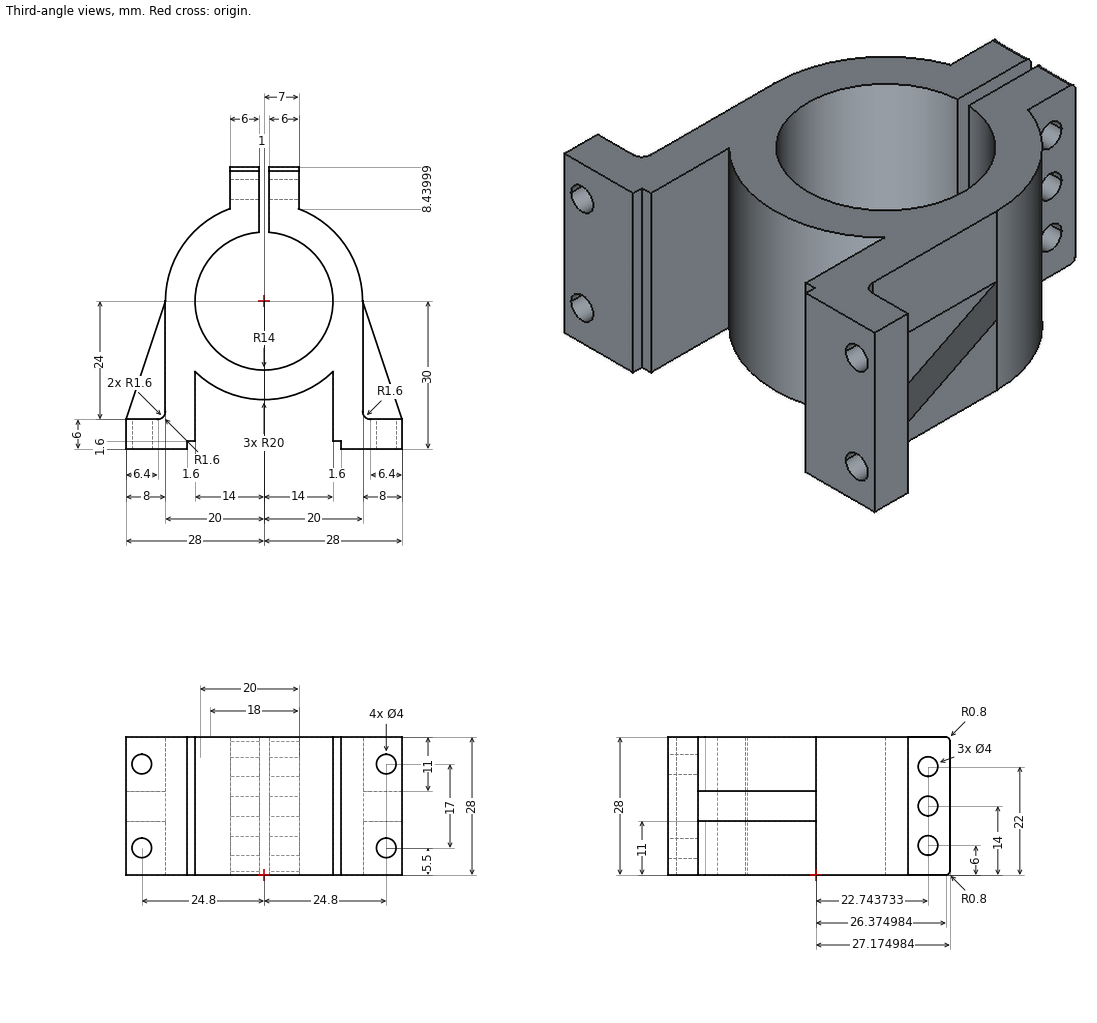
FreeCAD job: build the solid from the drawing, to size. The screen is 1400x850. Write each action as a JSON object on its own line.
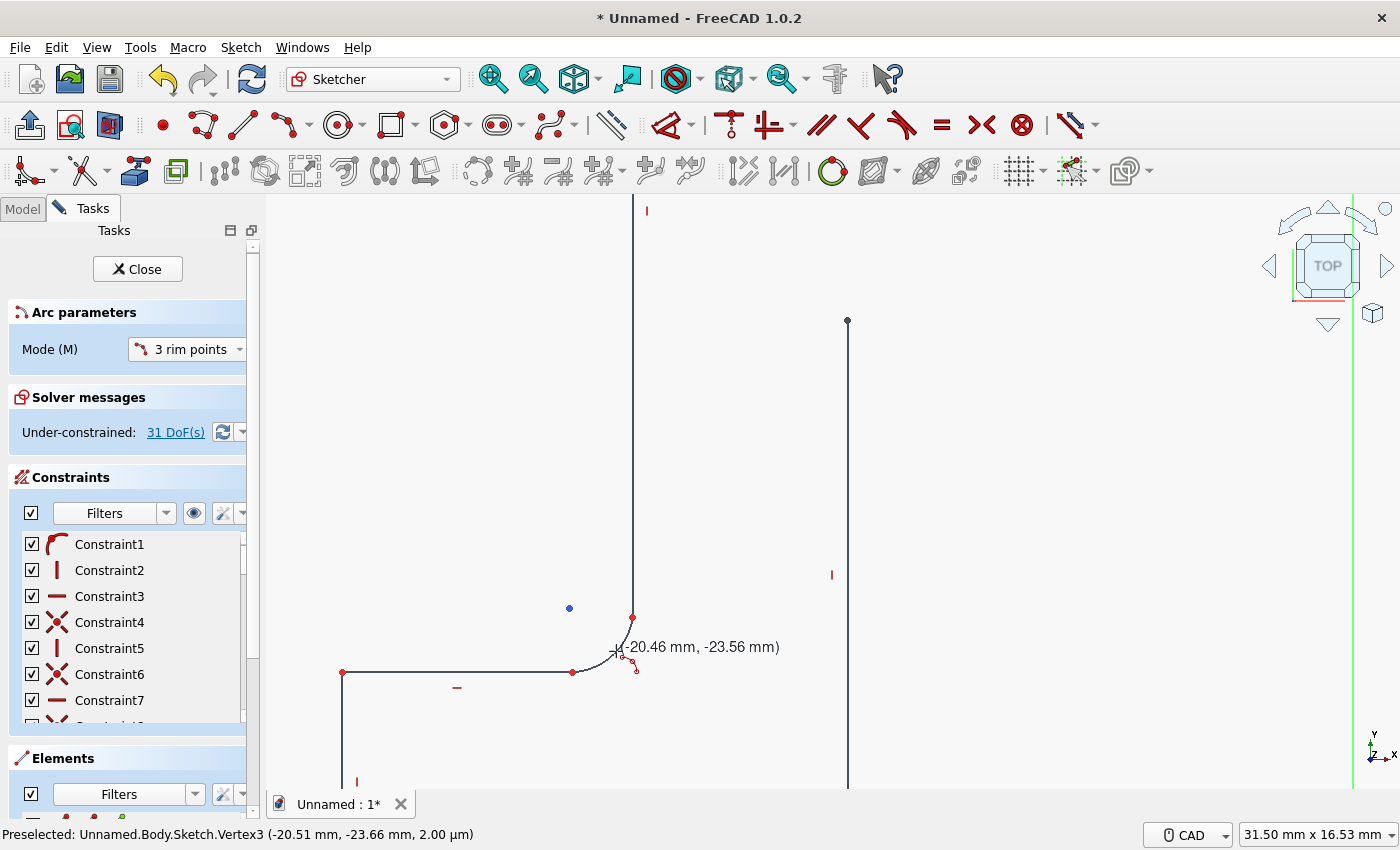
{"action": "scroll", "coordinate": [616, 653], "scroll_direction": "down", "scroll_amount": 8}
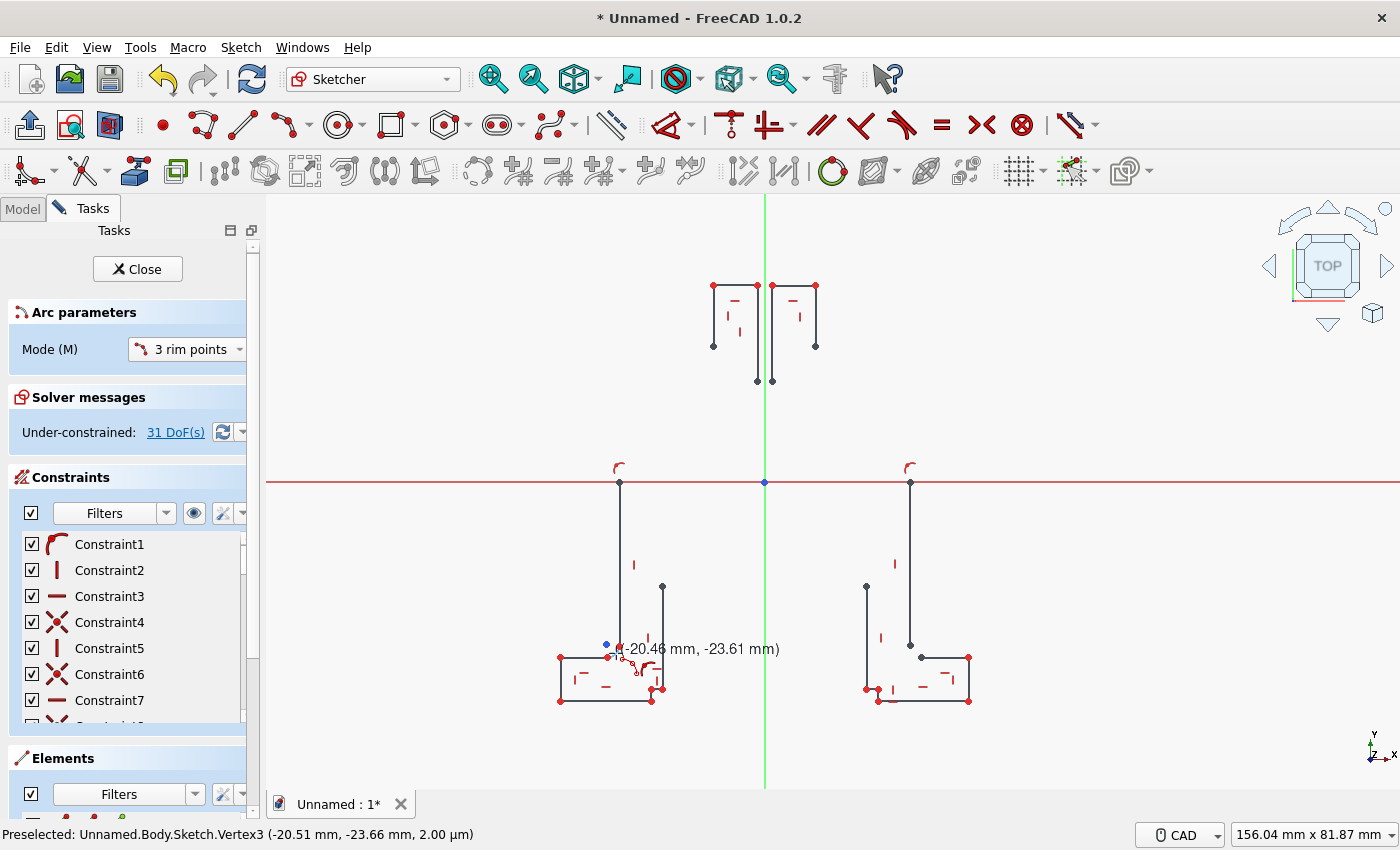
{"action": "left_click", "coordinate": [663, 587]}
{"action": "left_click", "coordinate": [867, 587]}
{"action": "left_click", "coordinate": [743, 626]}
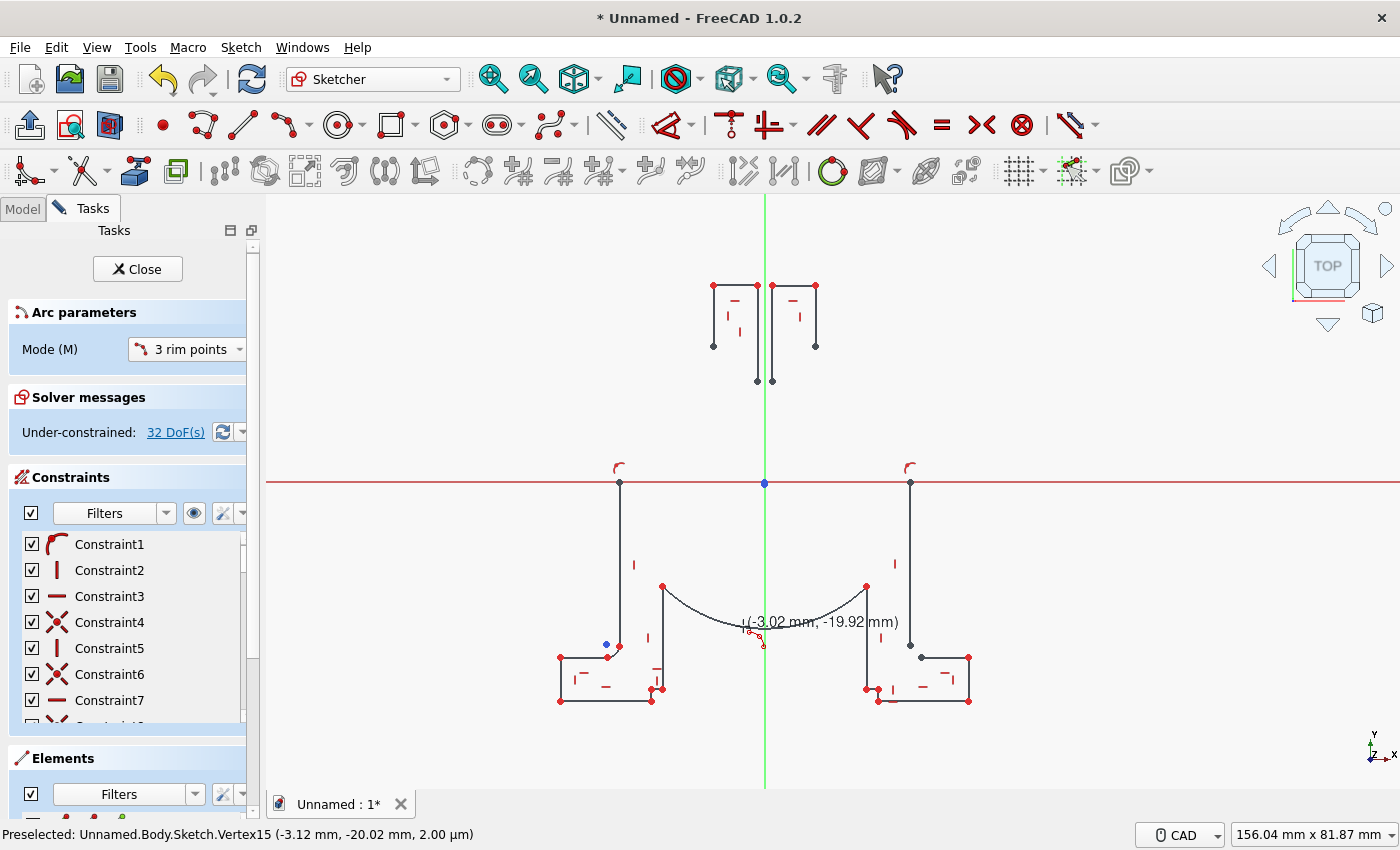
{"action": "left_click", "coordinate": [922, 658]}
{"action": "left_click", "coordinate": [910, 646]}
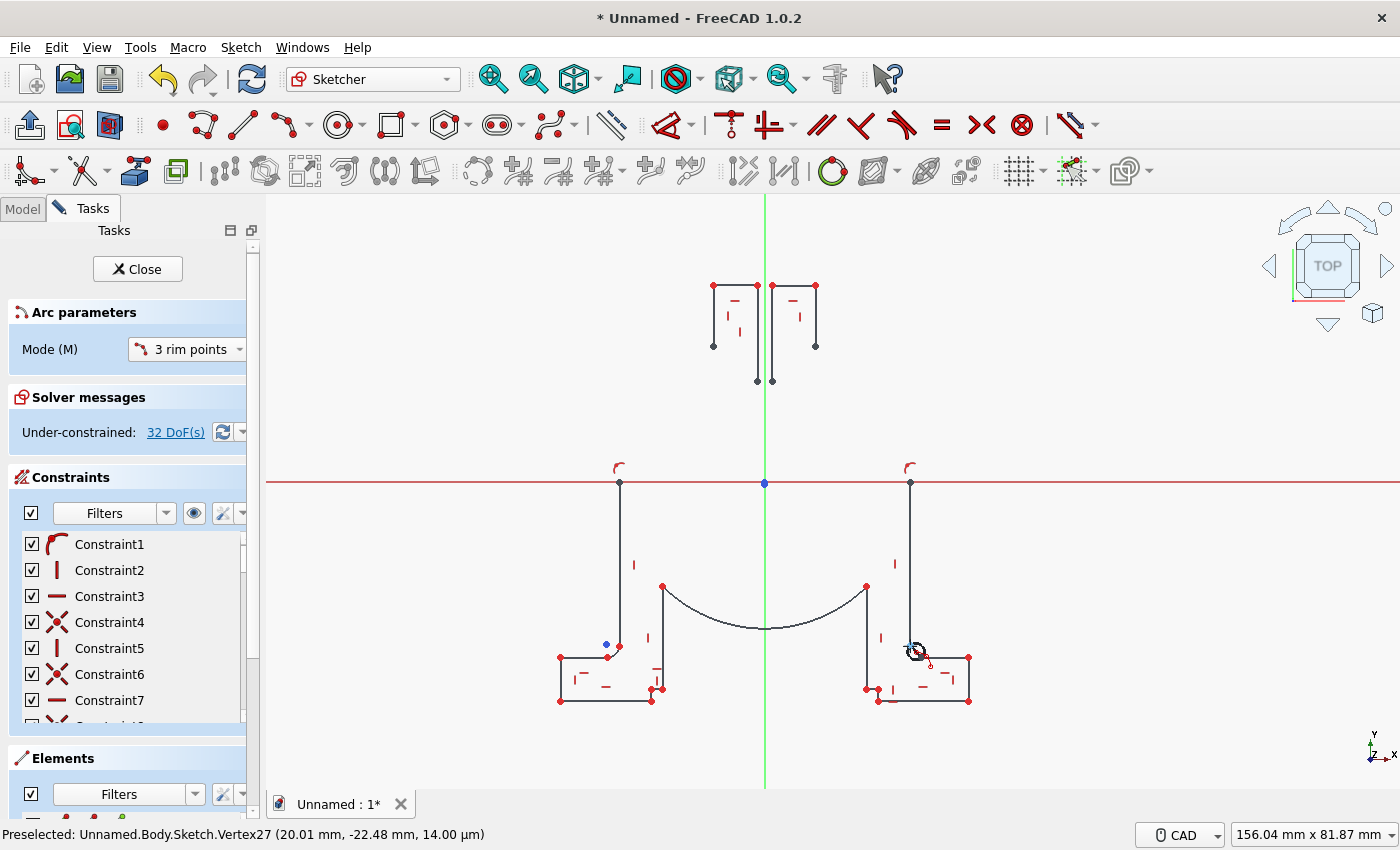
{"action": "scroll", "coordinate": [914, 653], "scroll_direction": "up", "scroll_amount": 8}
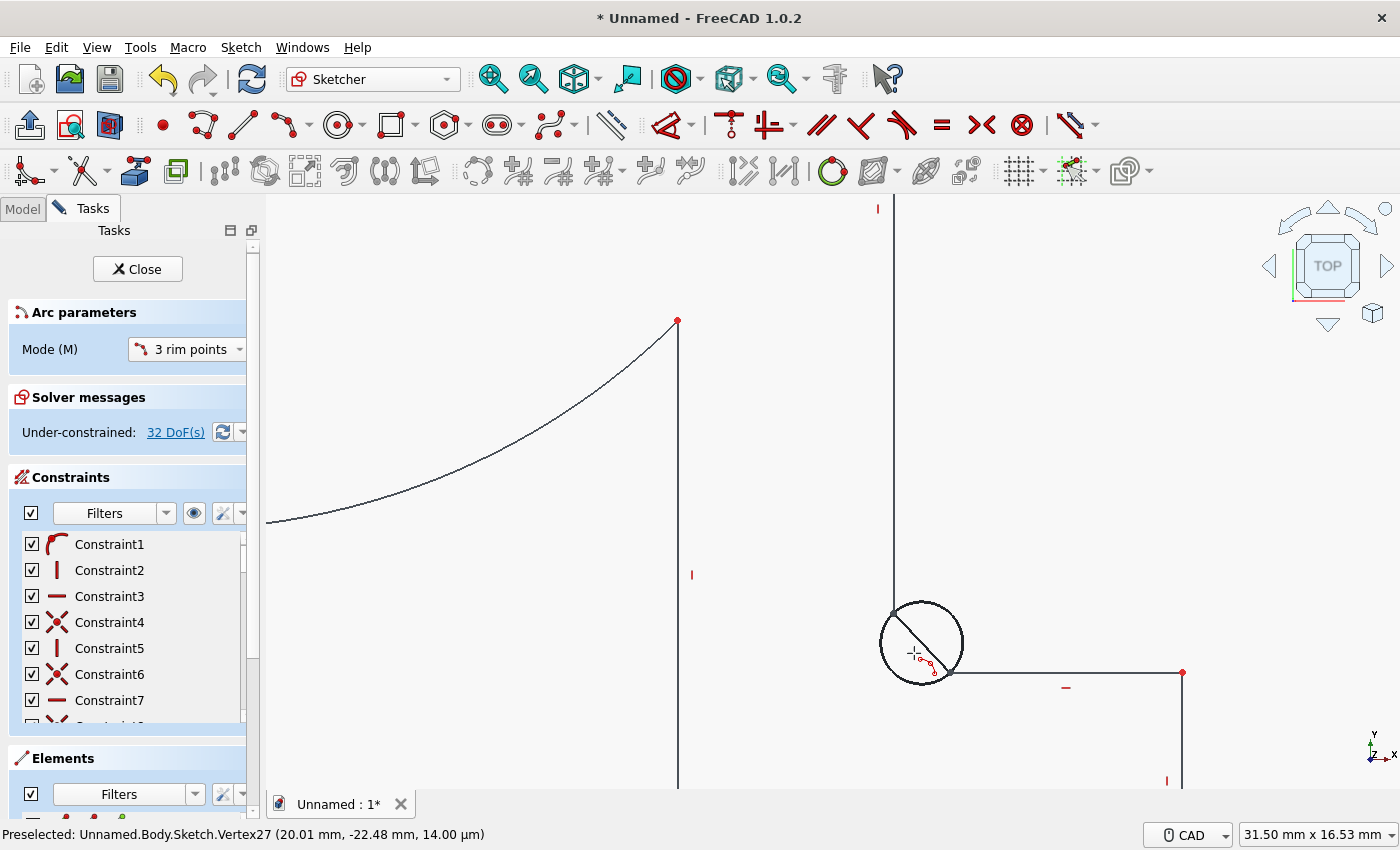
{"action": "left_click", "coordinate": [910, 651]}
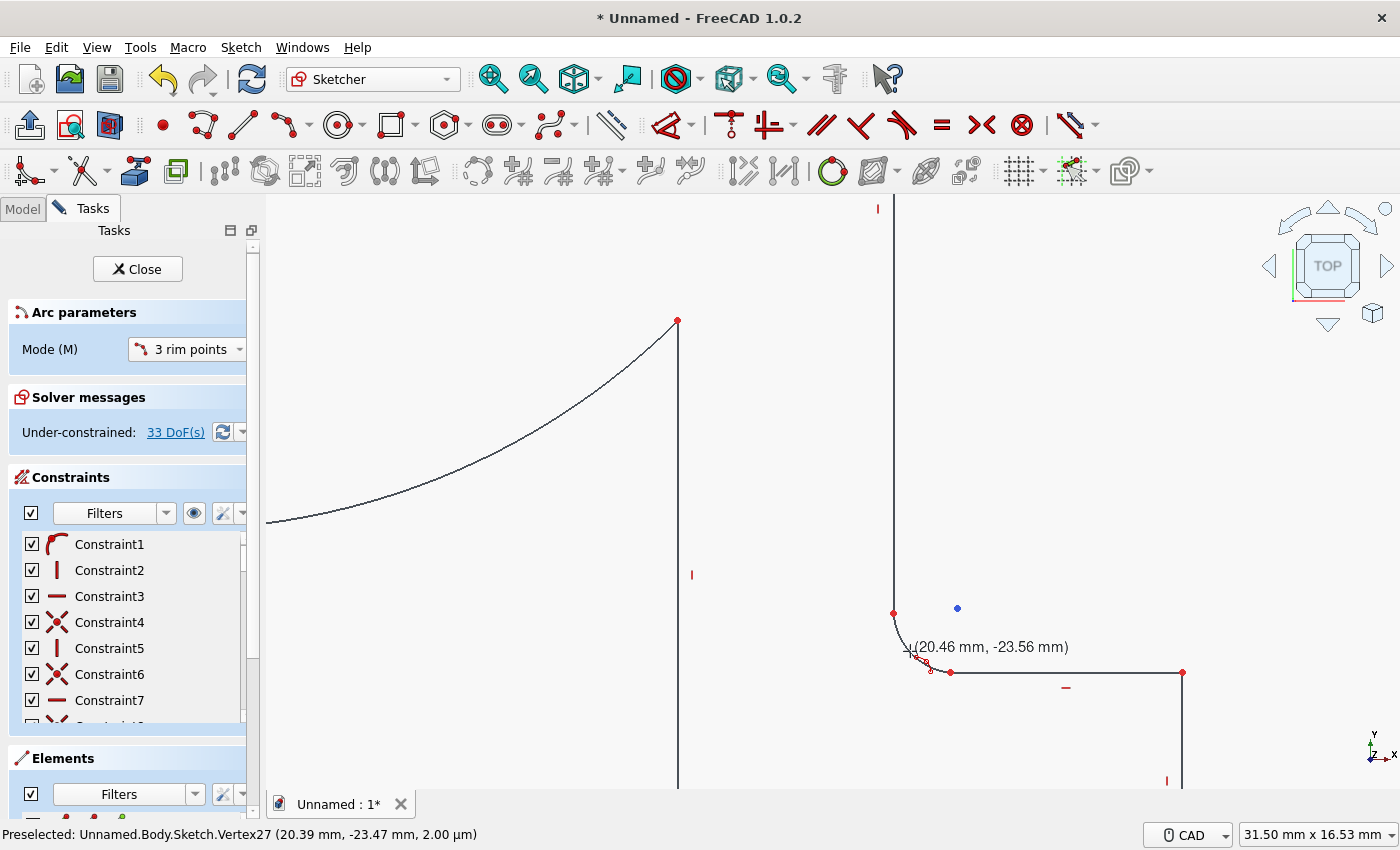
{"action": "scroll", "coordinate": [914, 653], "scroll_direction": "down", "scroll_amount": 8}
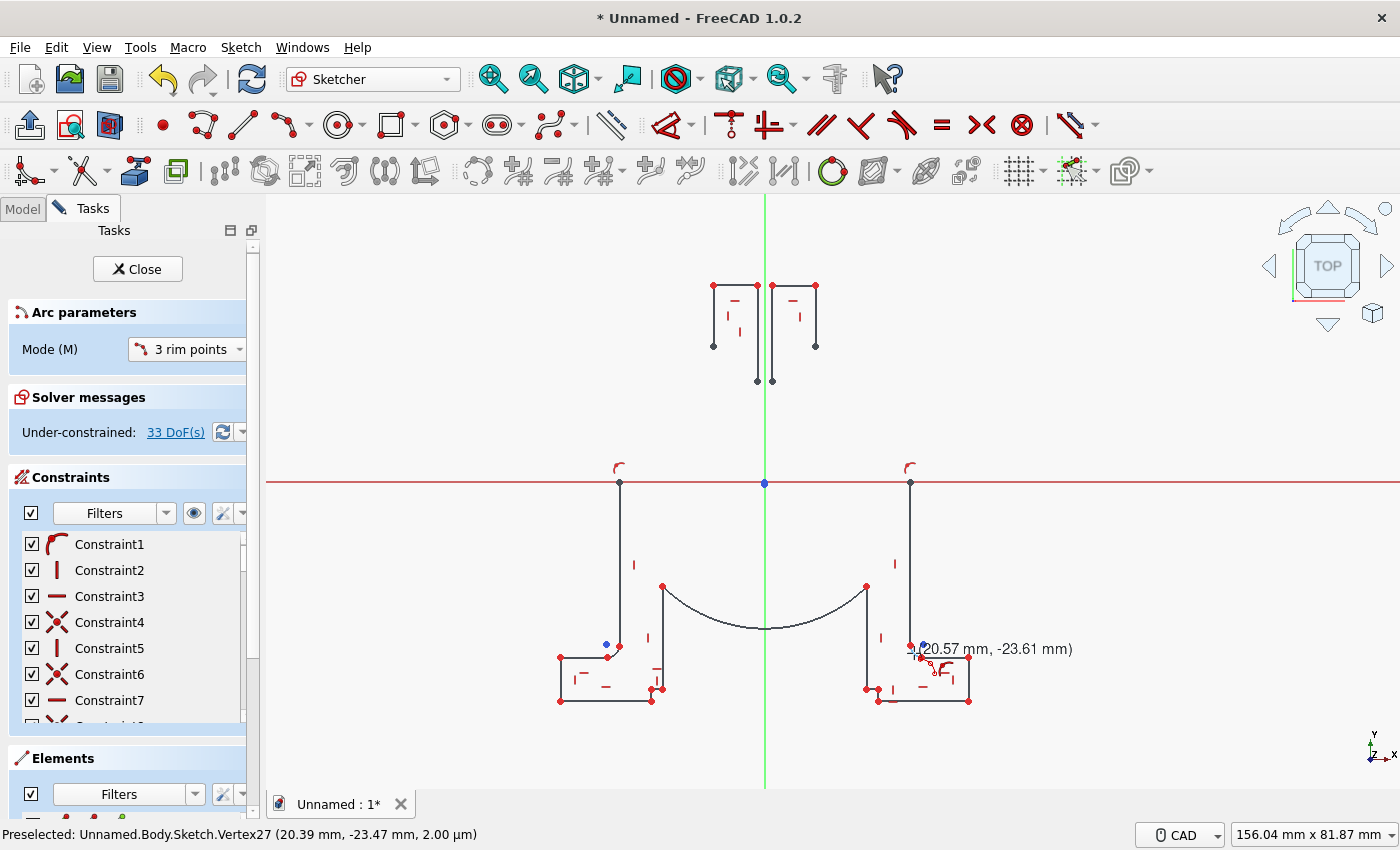
{"action": "left_click", "coordinate": [910, 482]}
{"action": "left_click", "coordinate": [816, 347]}
{"action": "left_click", "coordinate": [884, 399]}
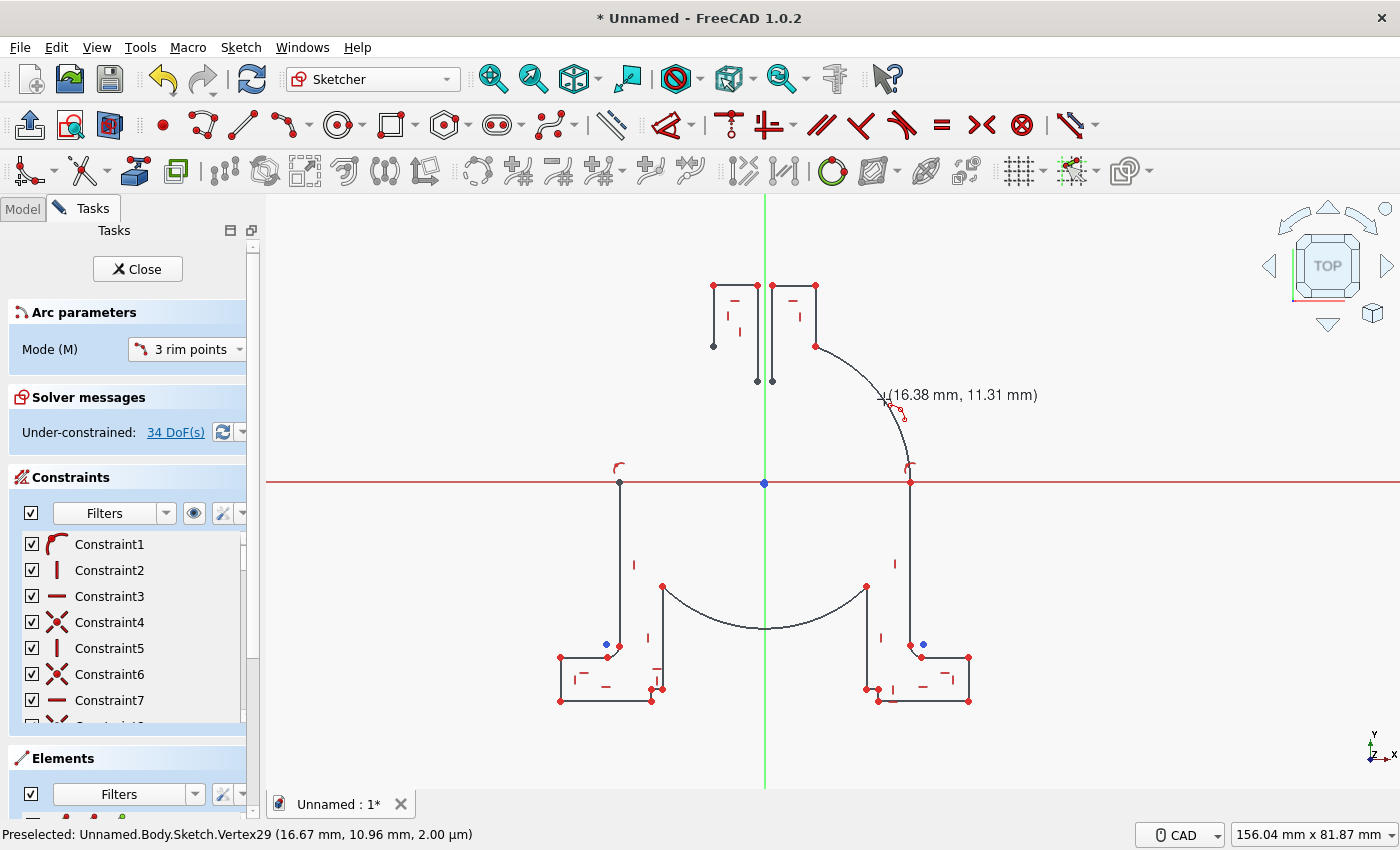
{"action": "scroll", "coordinate": [772, 381], "scroll_direction": "up", "scroll_amount": 4}